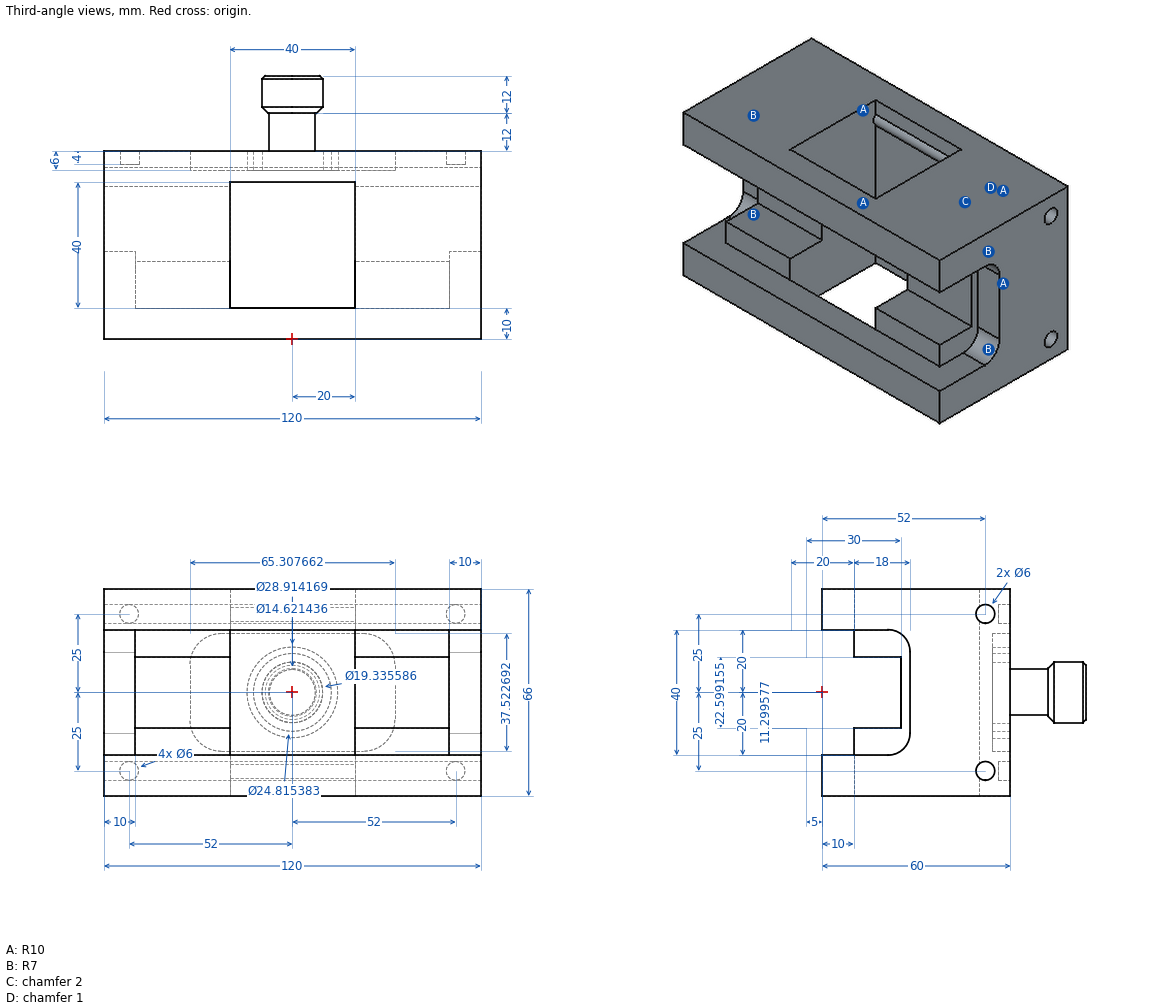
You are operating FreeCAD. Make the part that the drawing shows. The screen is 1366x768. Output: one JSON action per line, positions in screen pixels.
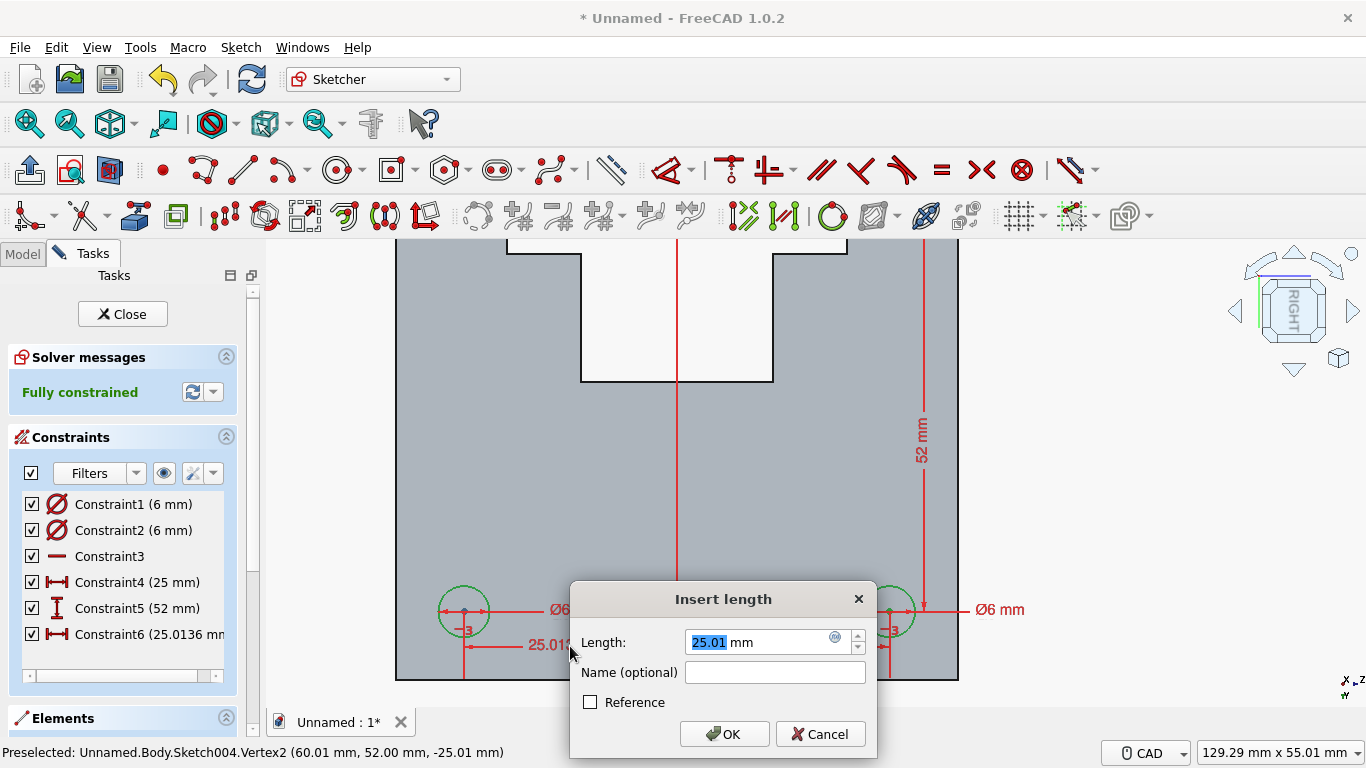
{"action": "type", "text": "25"}
{"action": "key", "text": "Return"}
{"action": "key", "text": "Escape"}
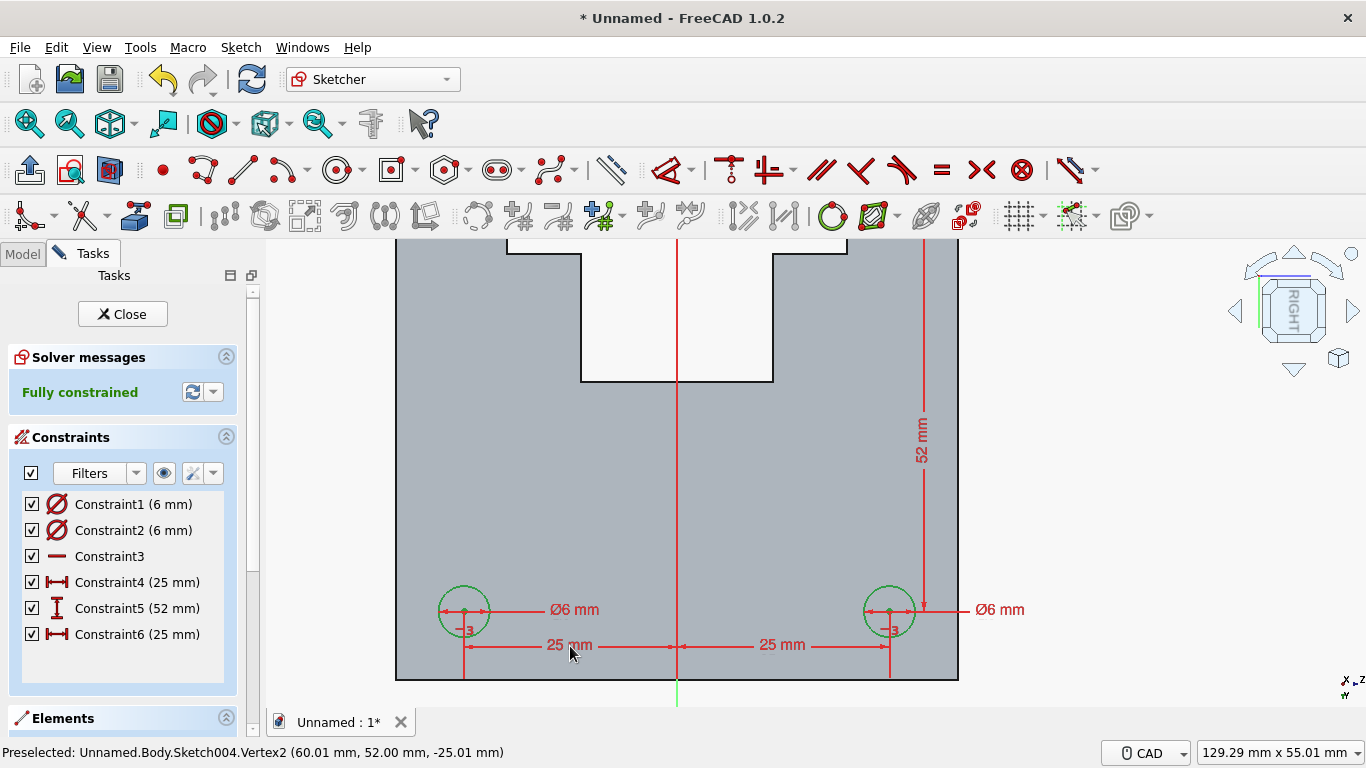
{"action": "left_click", "coordinate": [123, 314]}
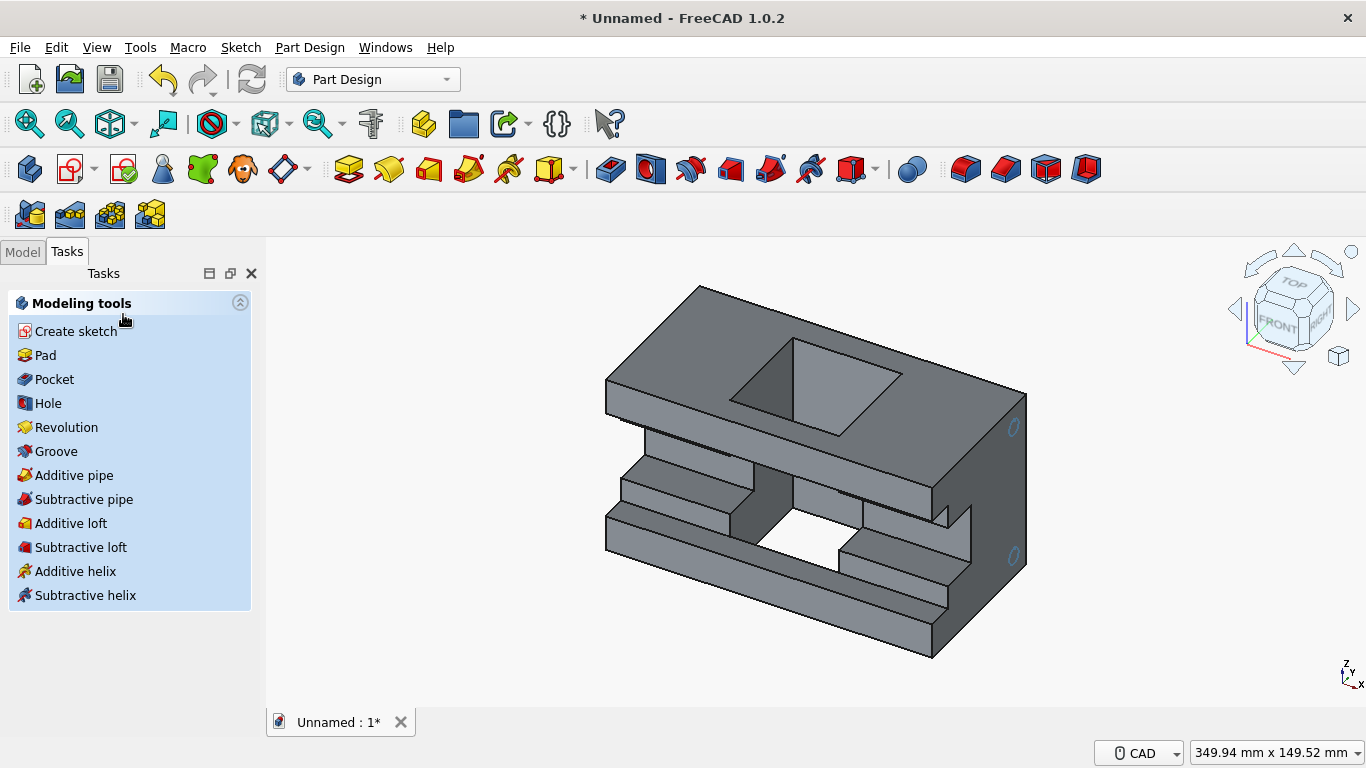
{"action": "left_click", "coordinate": [612, 170]}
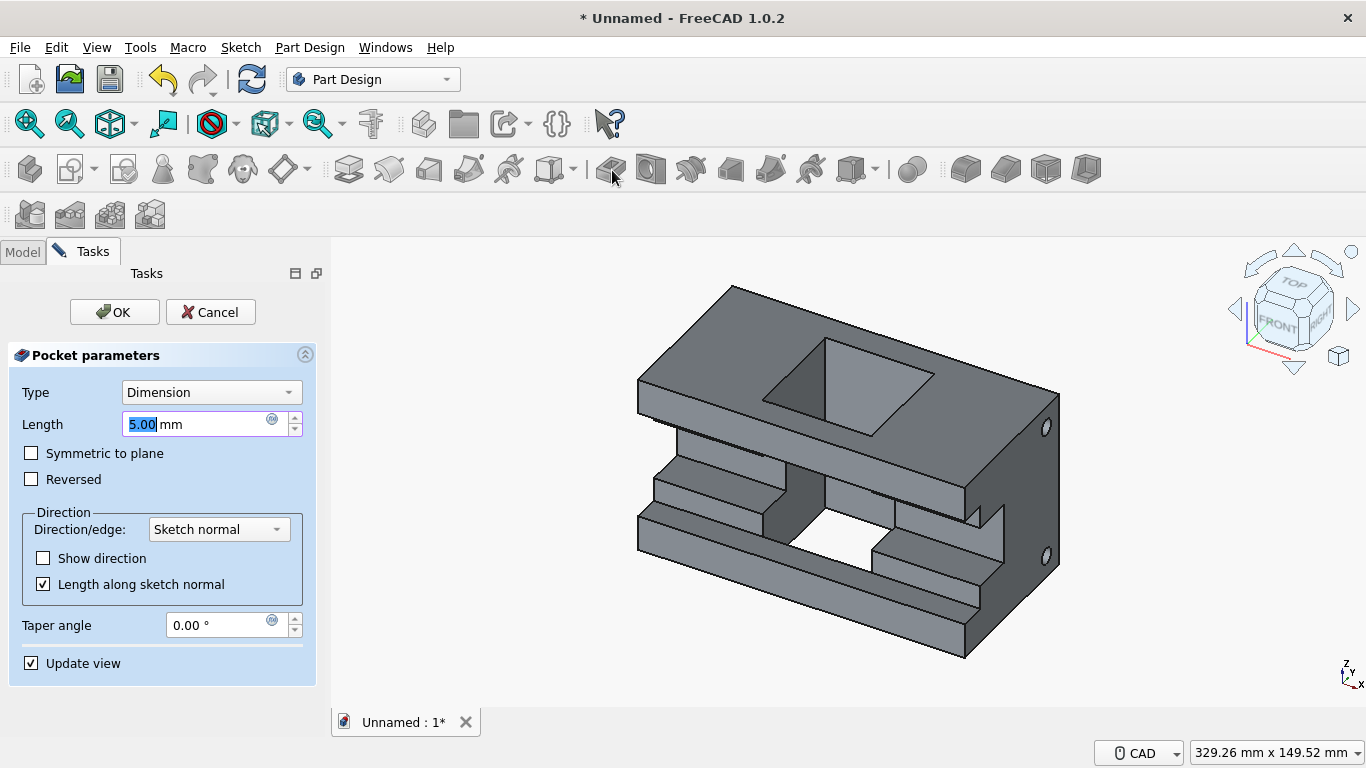
{"action": "type", "text": "120"}
{"action": "key", "text": "Tab"}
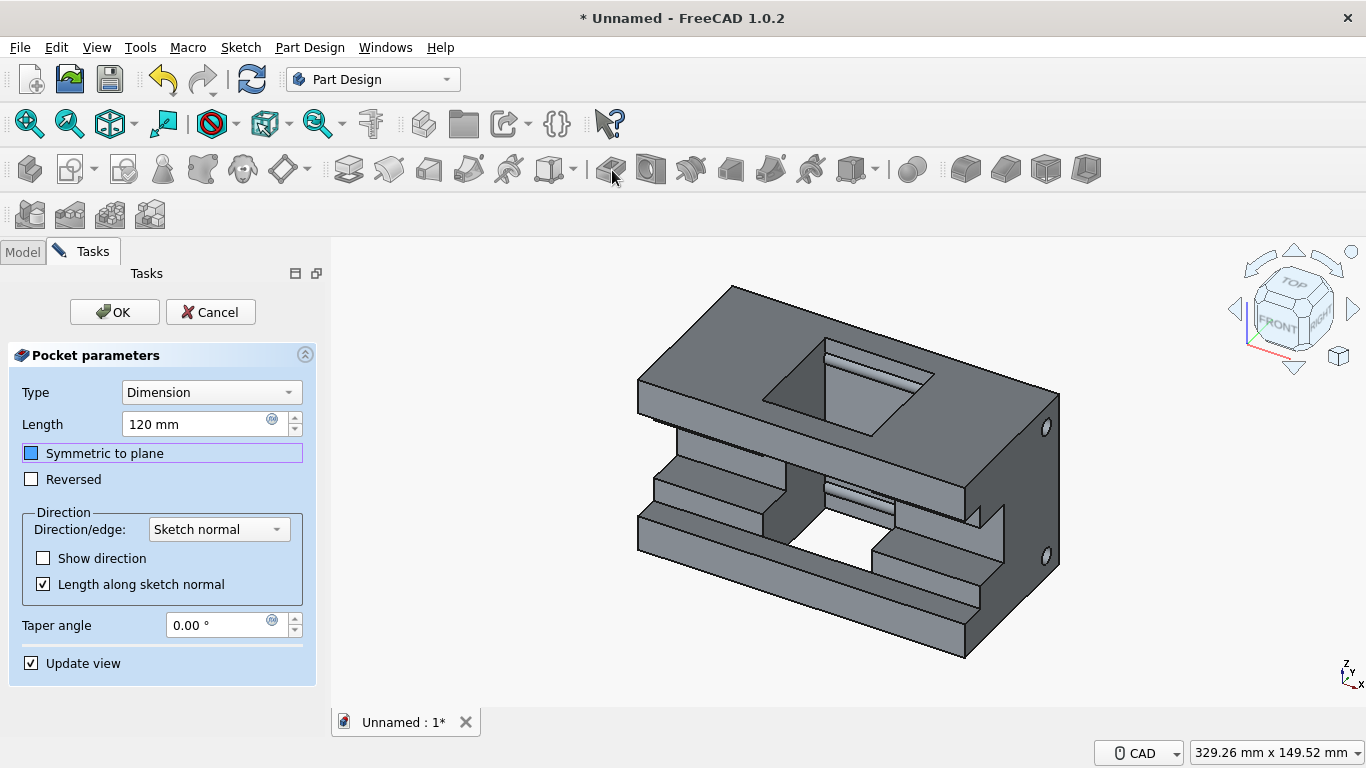
{"action": "left_click", "coordinate": [115, 312]}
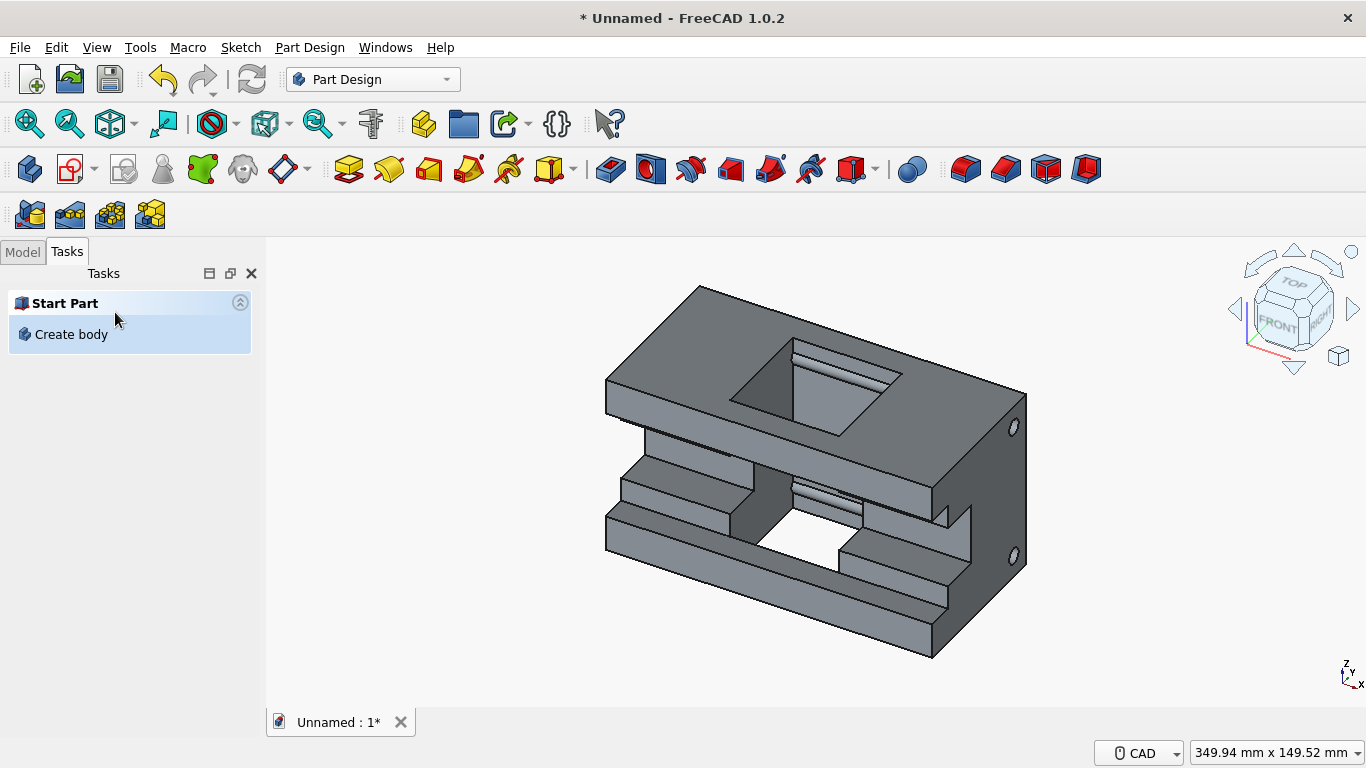
{"action": "left_click", "coordinate": [993, 487]}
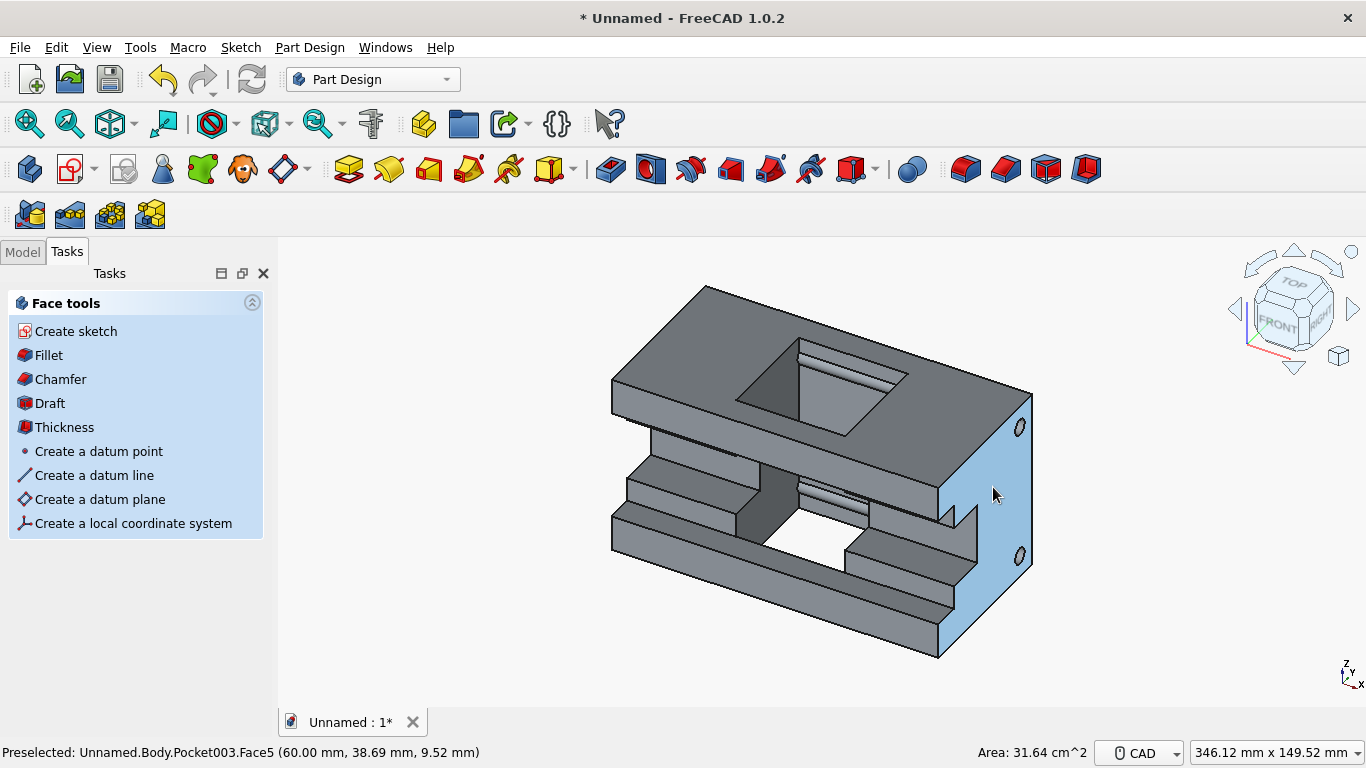
{"action": "left_click", "coordinate": [70, 170]}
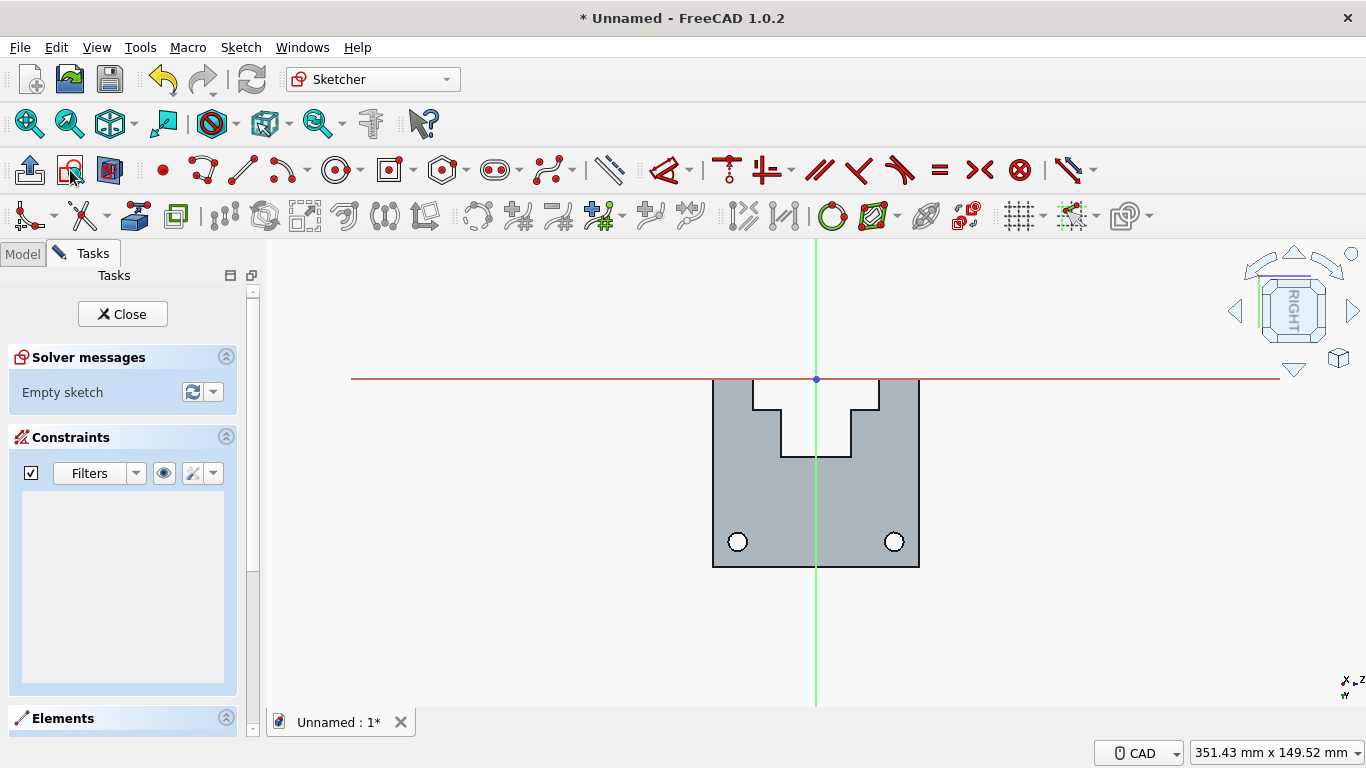
{"action": "scroll", "coordinate": [846, 401], "scroll_direction": "up", "scroll_amount": 6}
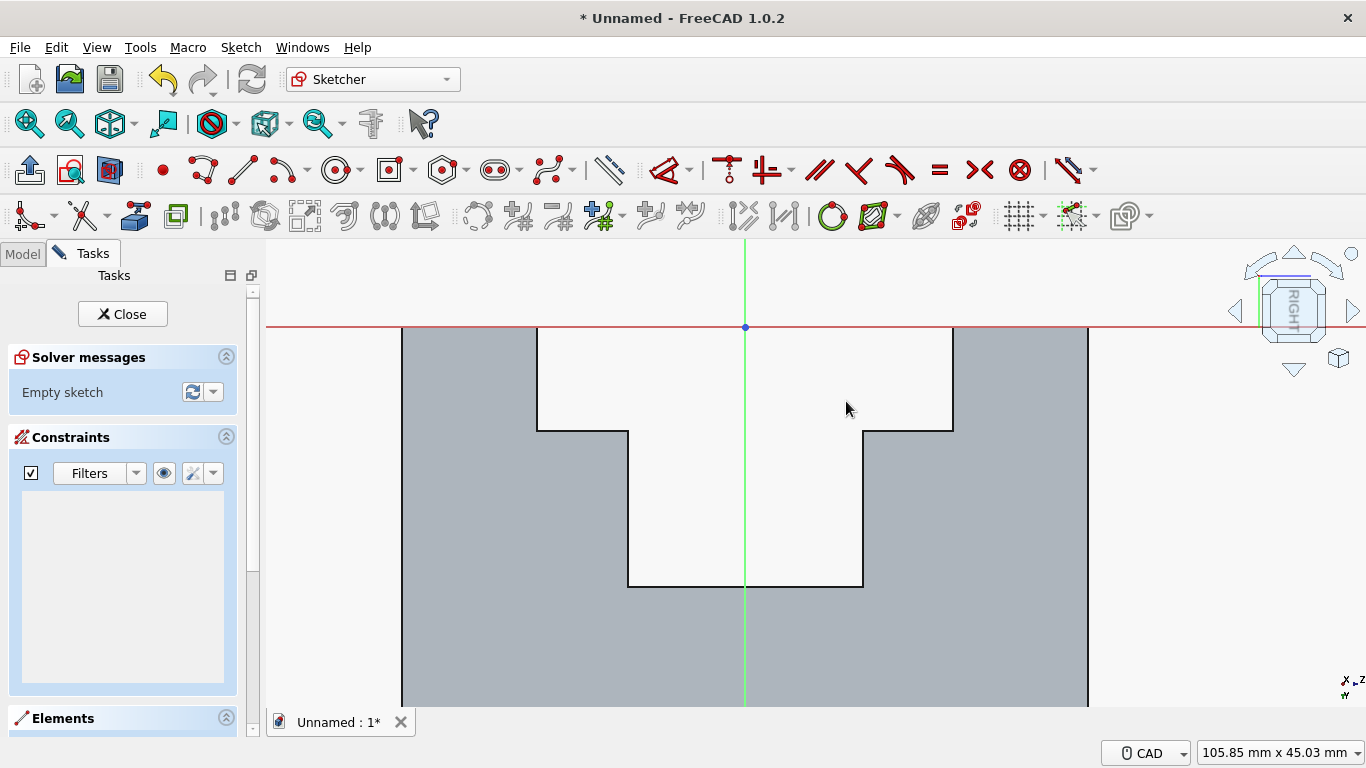
{"action": "key", "text": "g r"}